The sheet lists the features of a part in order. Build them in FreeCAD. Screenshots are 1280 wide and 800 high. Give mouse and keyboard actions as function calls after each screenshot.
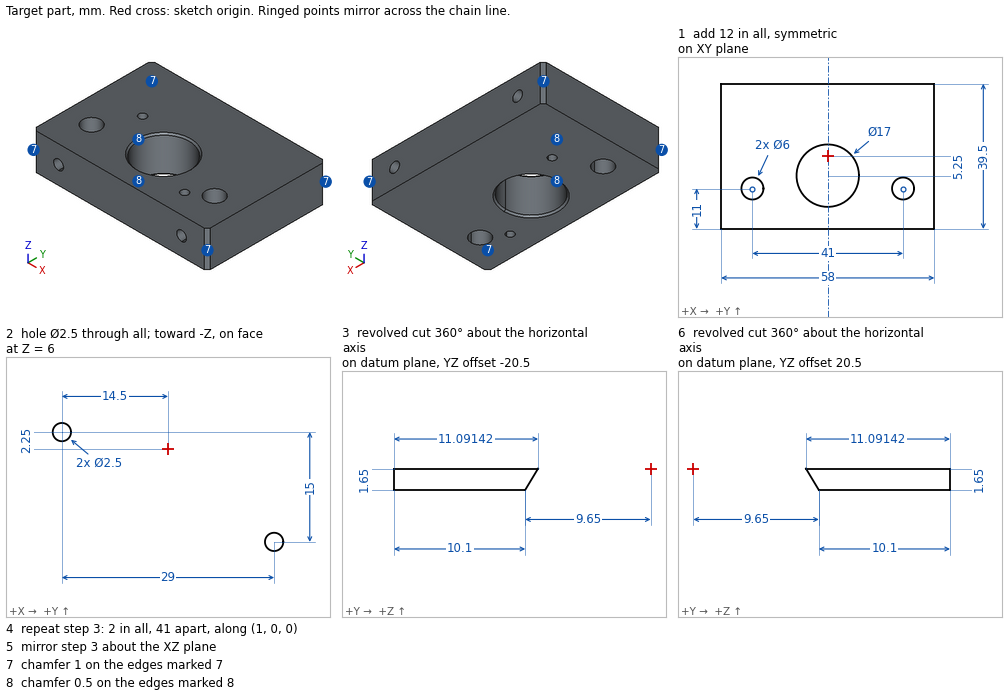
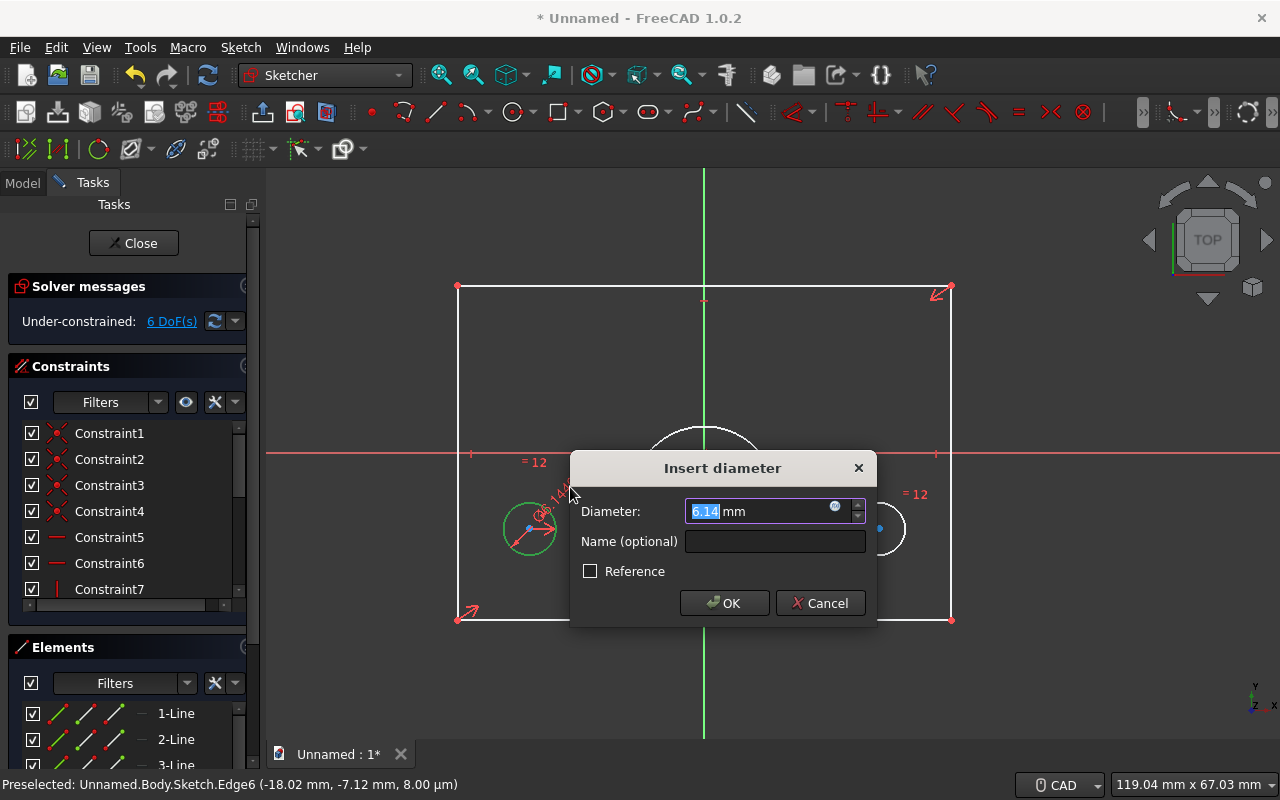
text(6)
key(Return)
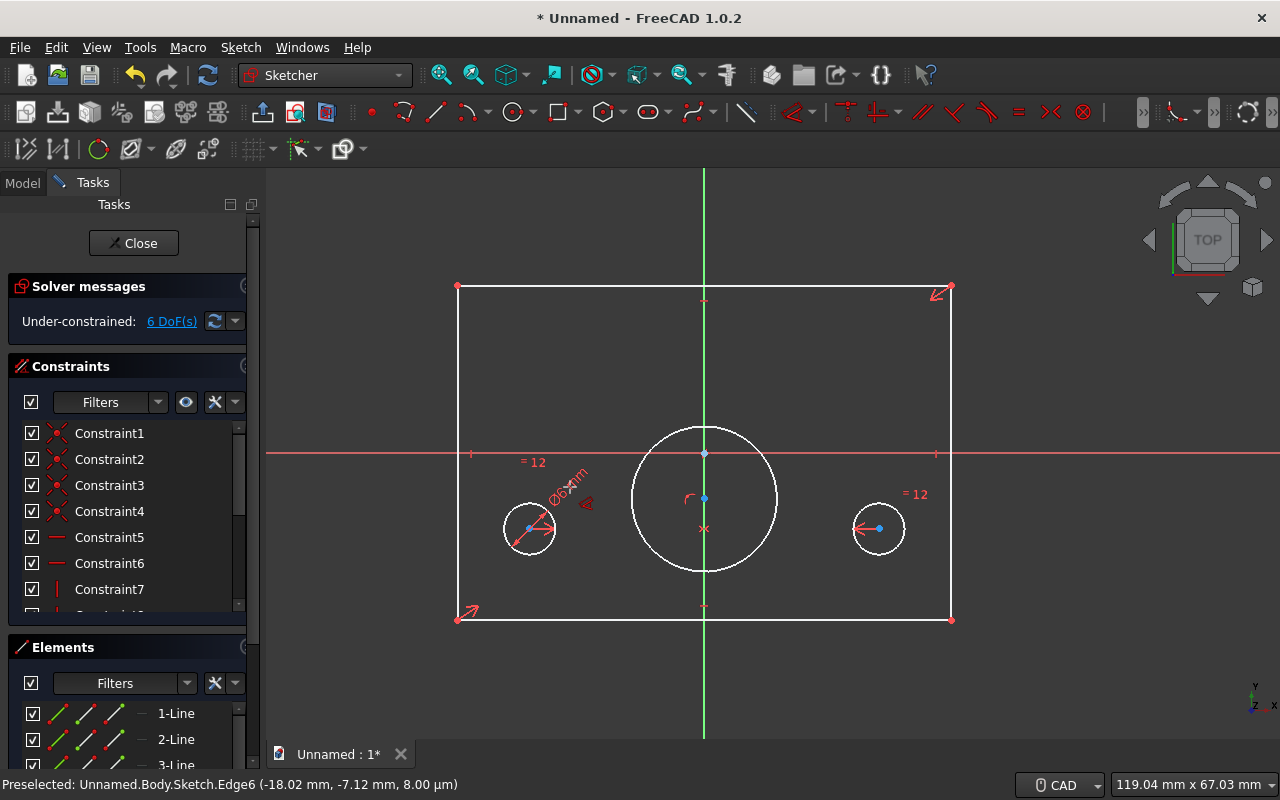
click(653, 550)
click(630, 573)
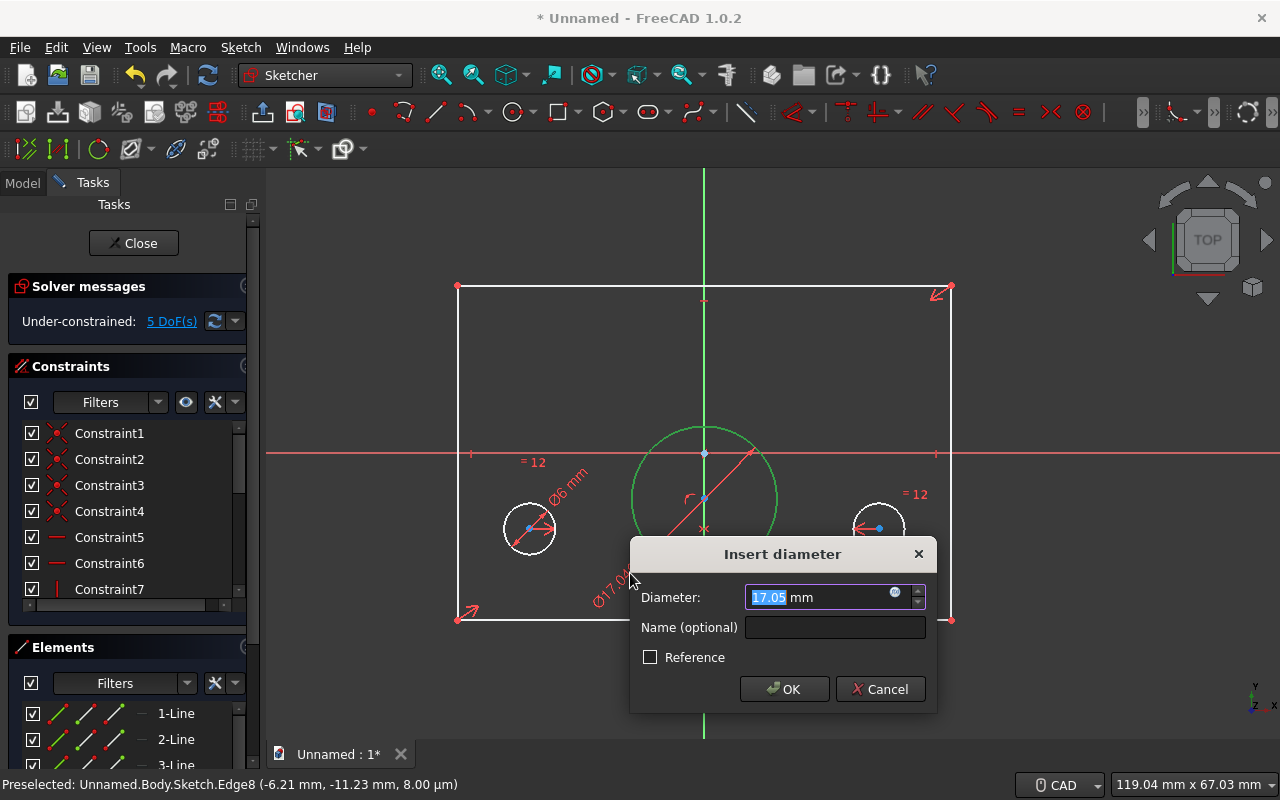
text(17)
key(Return)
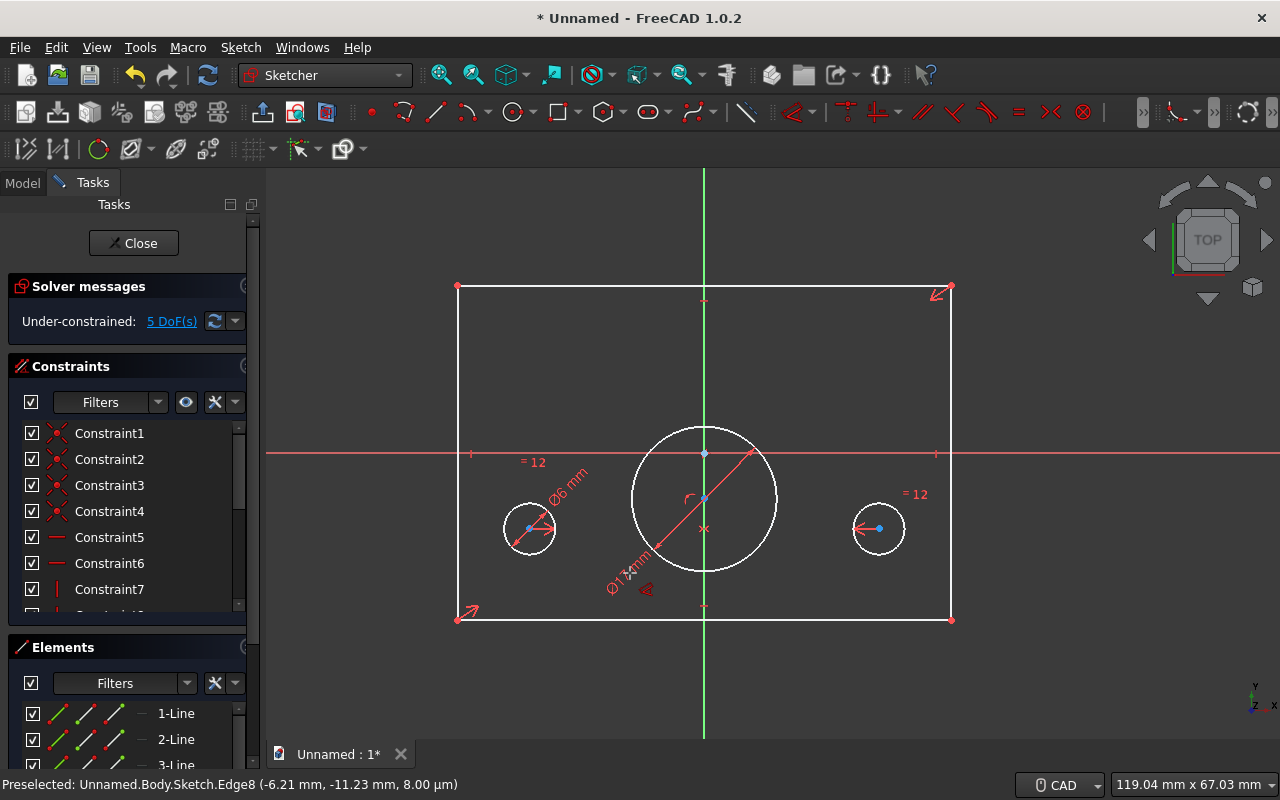
click(606, 620)
click(591, 654)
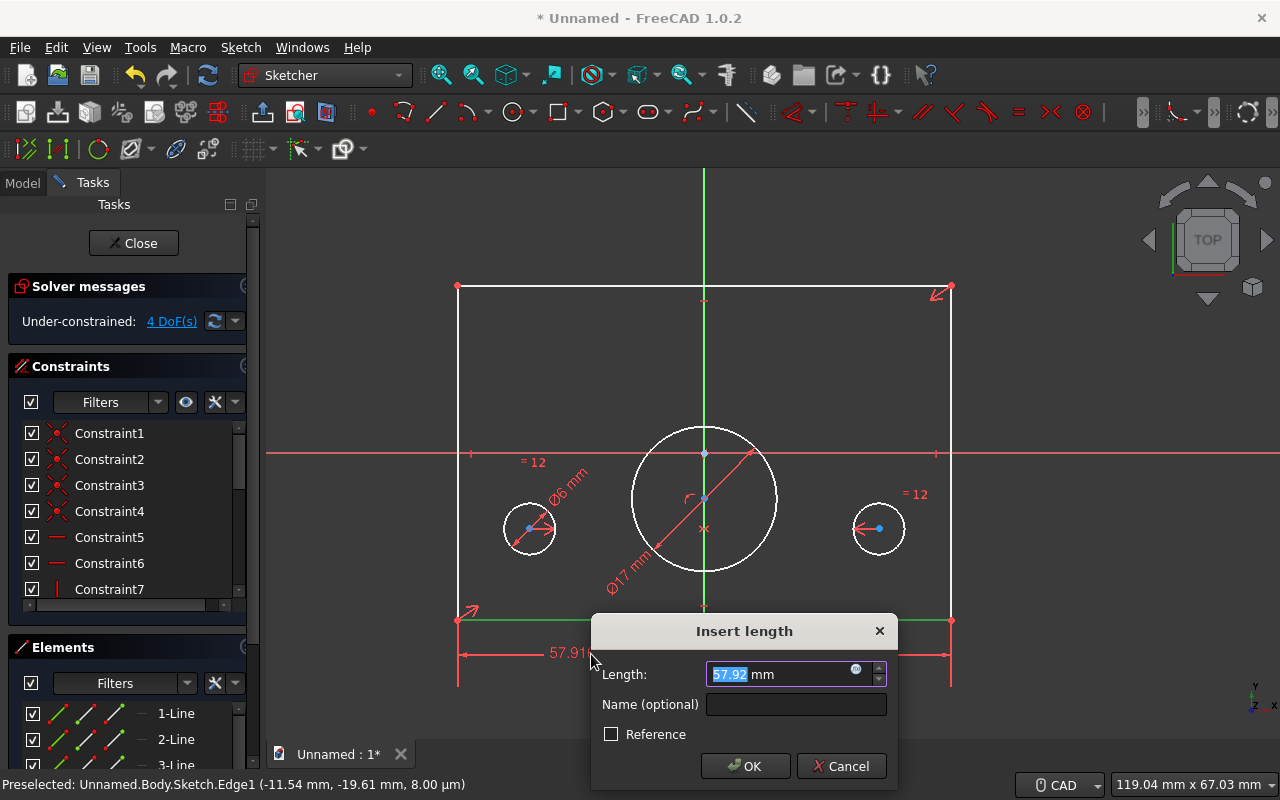
text(58)
key(Return)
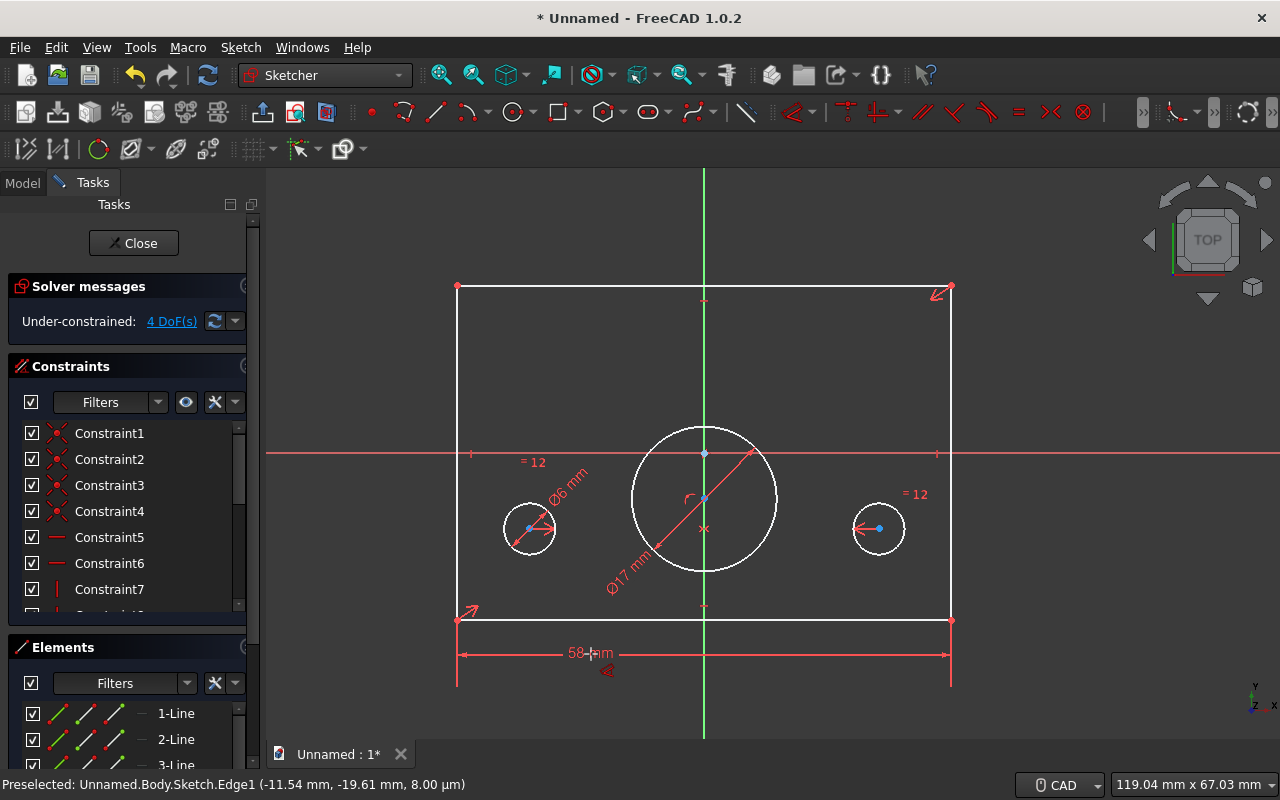
click(457, 620)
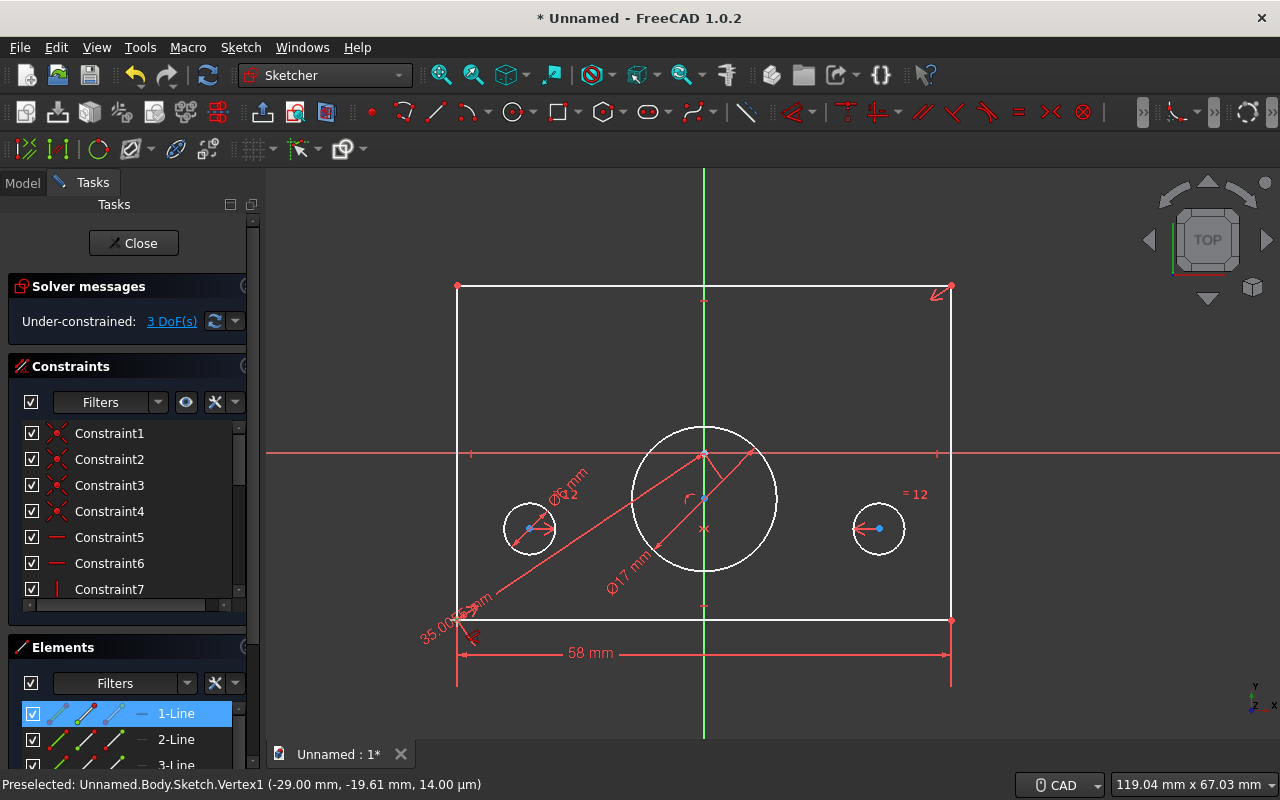
click(530, 529)
click(423, 575)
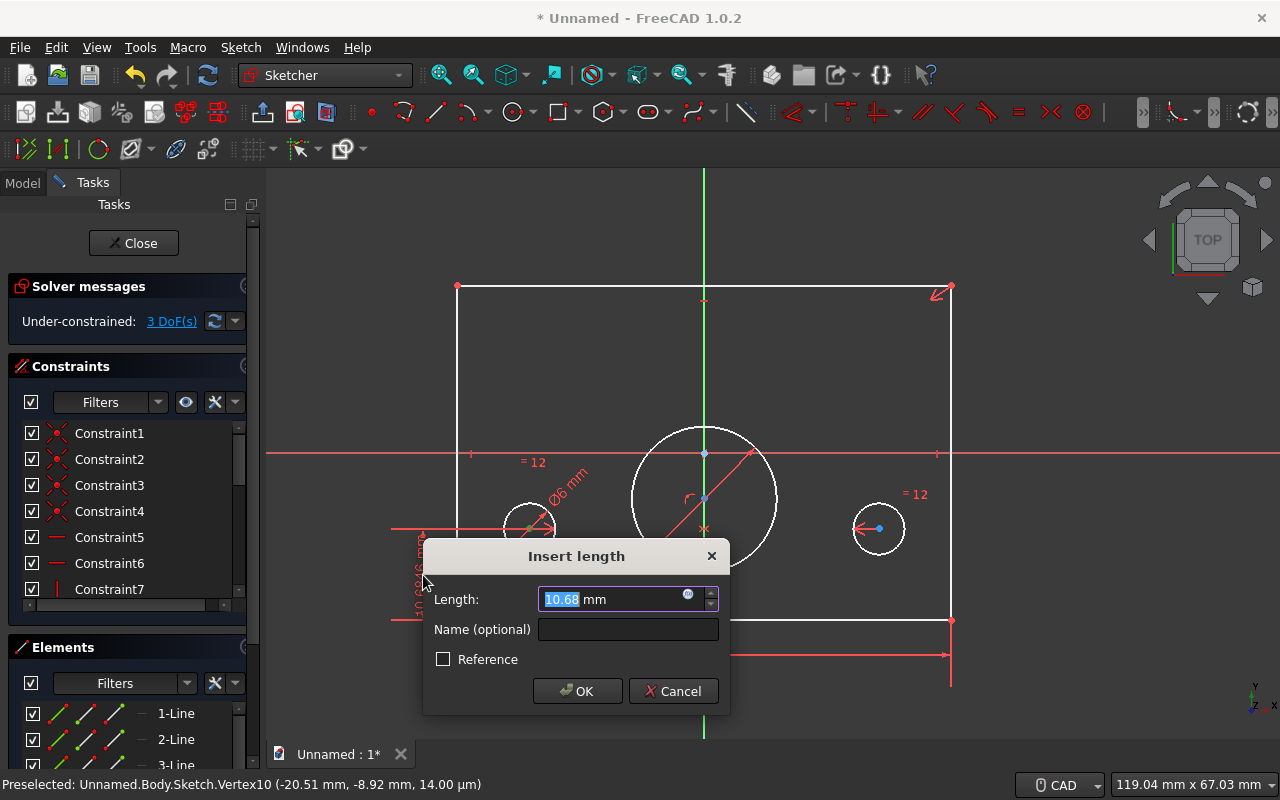
text(11)
key(Return)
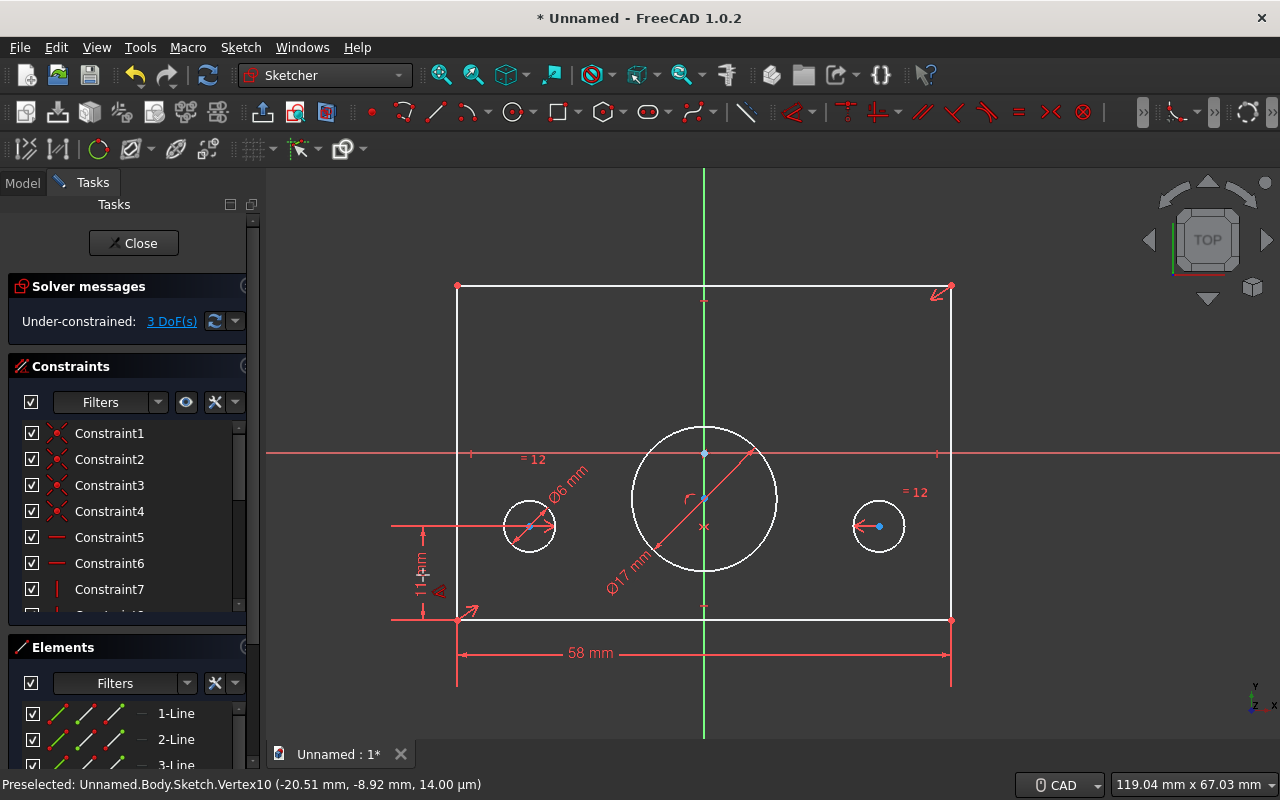
click(530, 526)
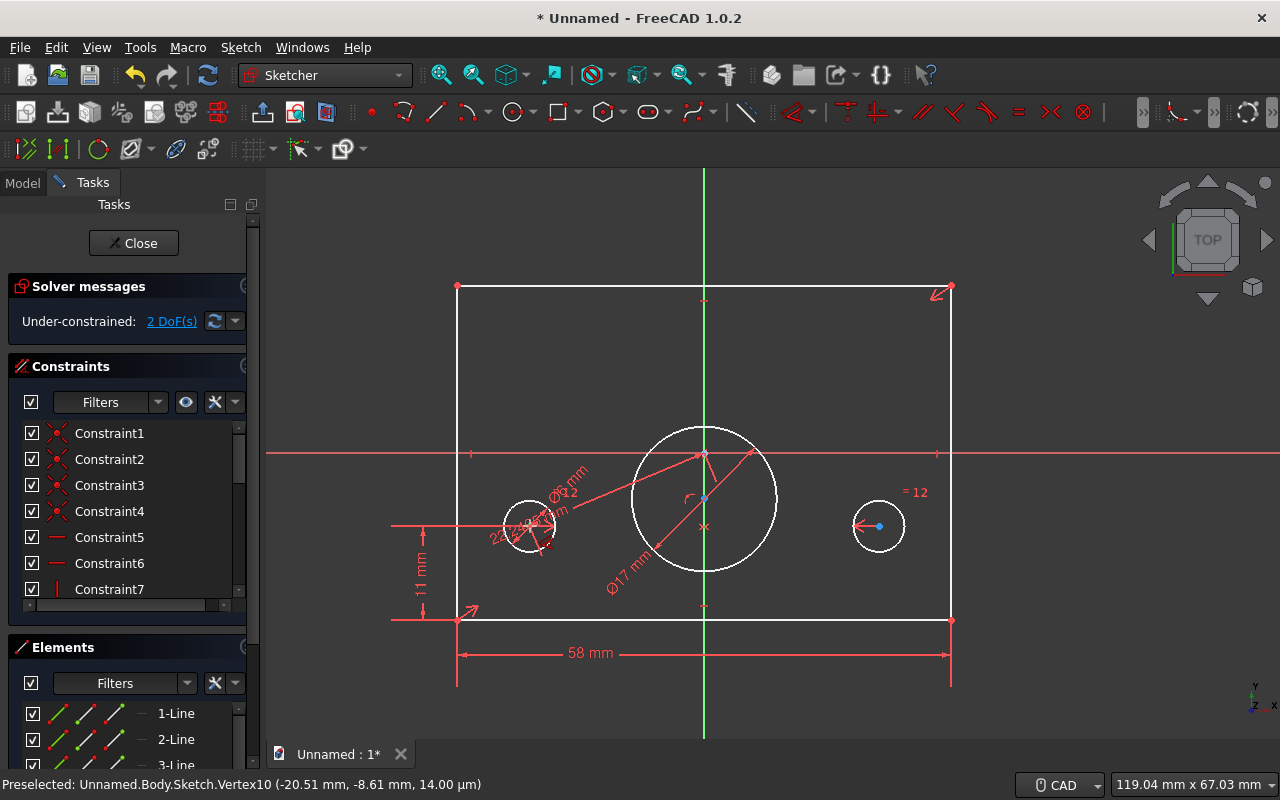
click(879, 526)
click(785, 560)